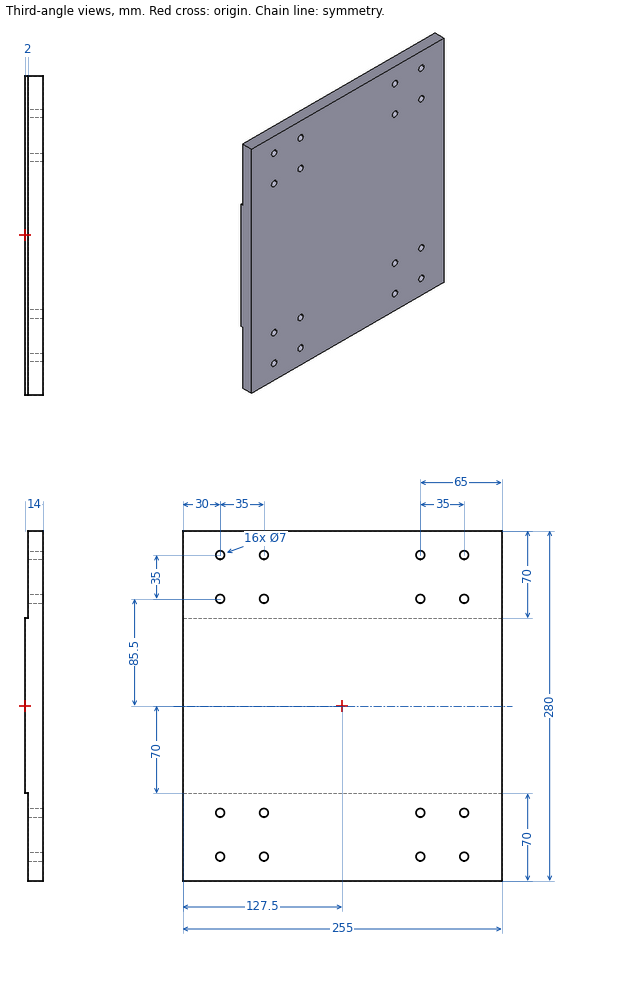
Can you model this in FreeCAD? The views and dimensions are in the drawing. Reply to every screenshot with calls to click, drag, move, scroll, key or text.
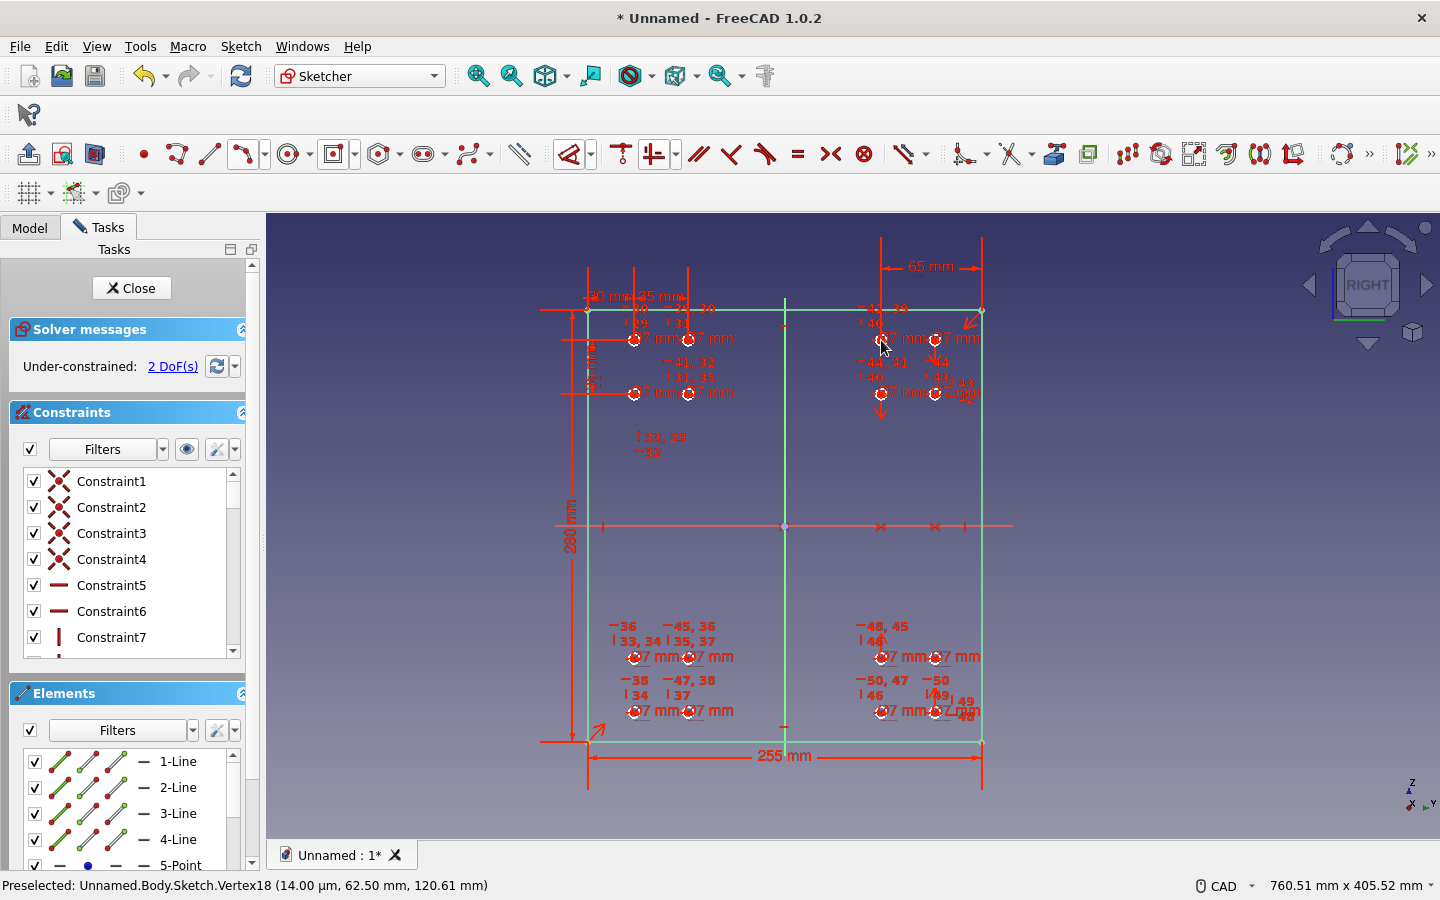
click(935, 340)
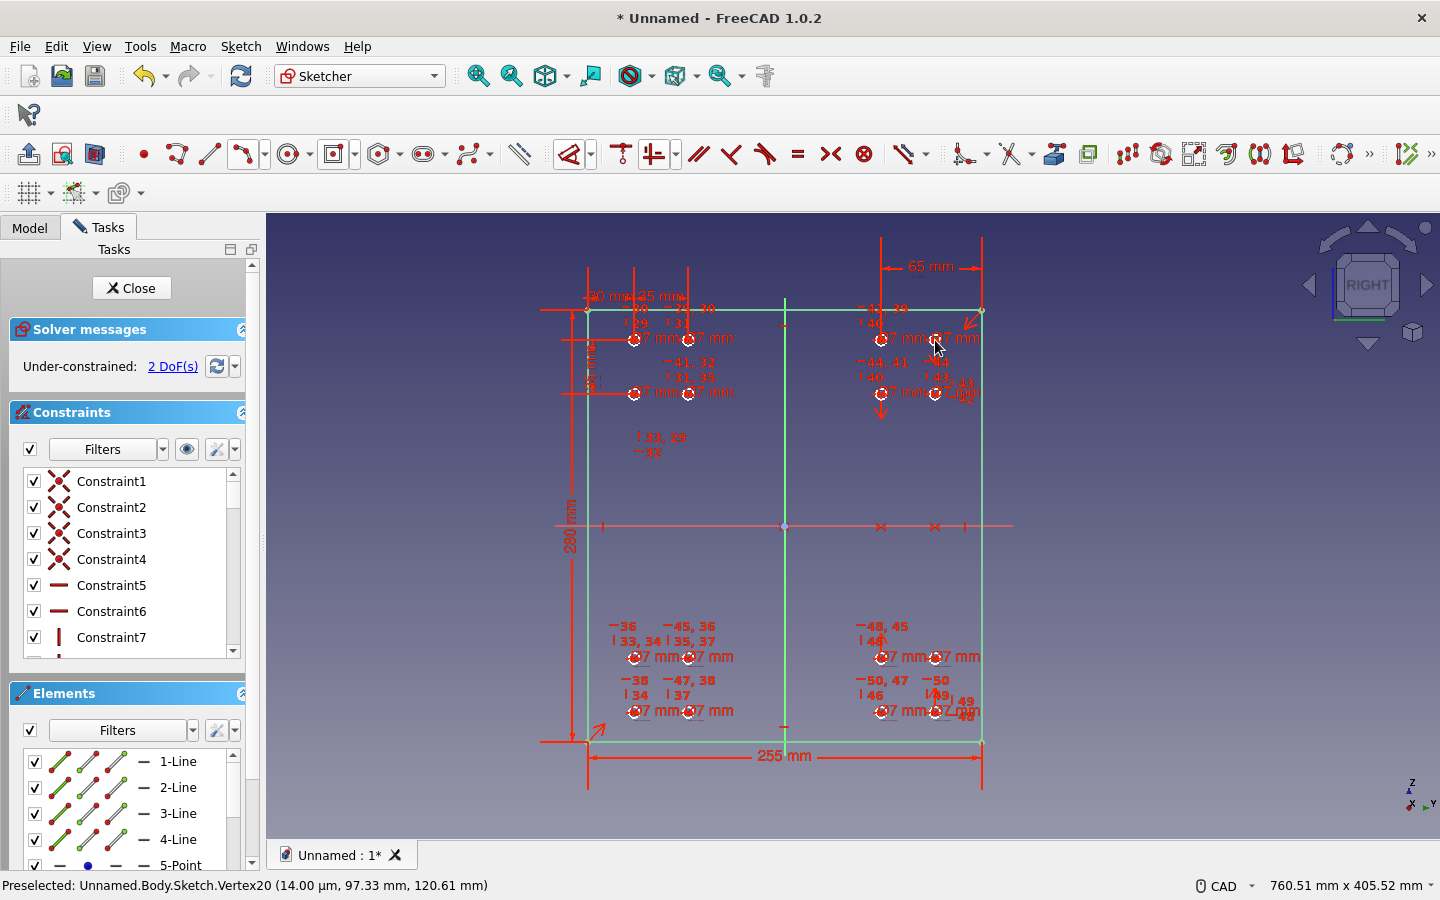
click(590, 154)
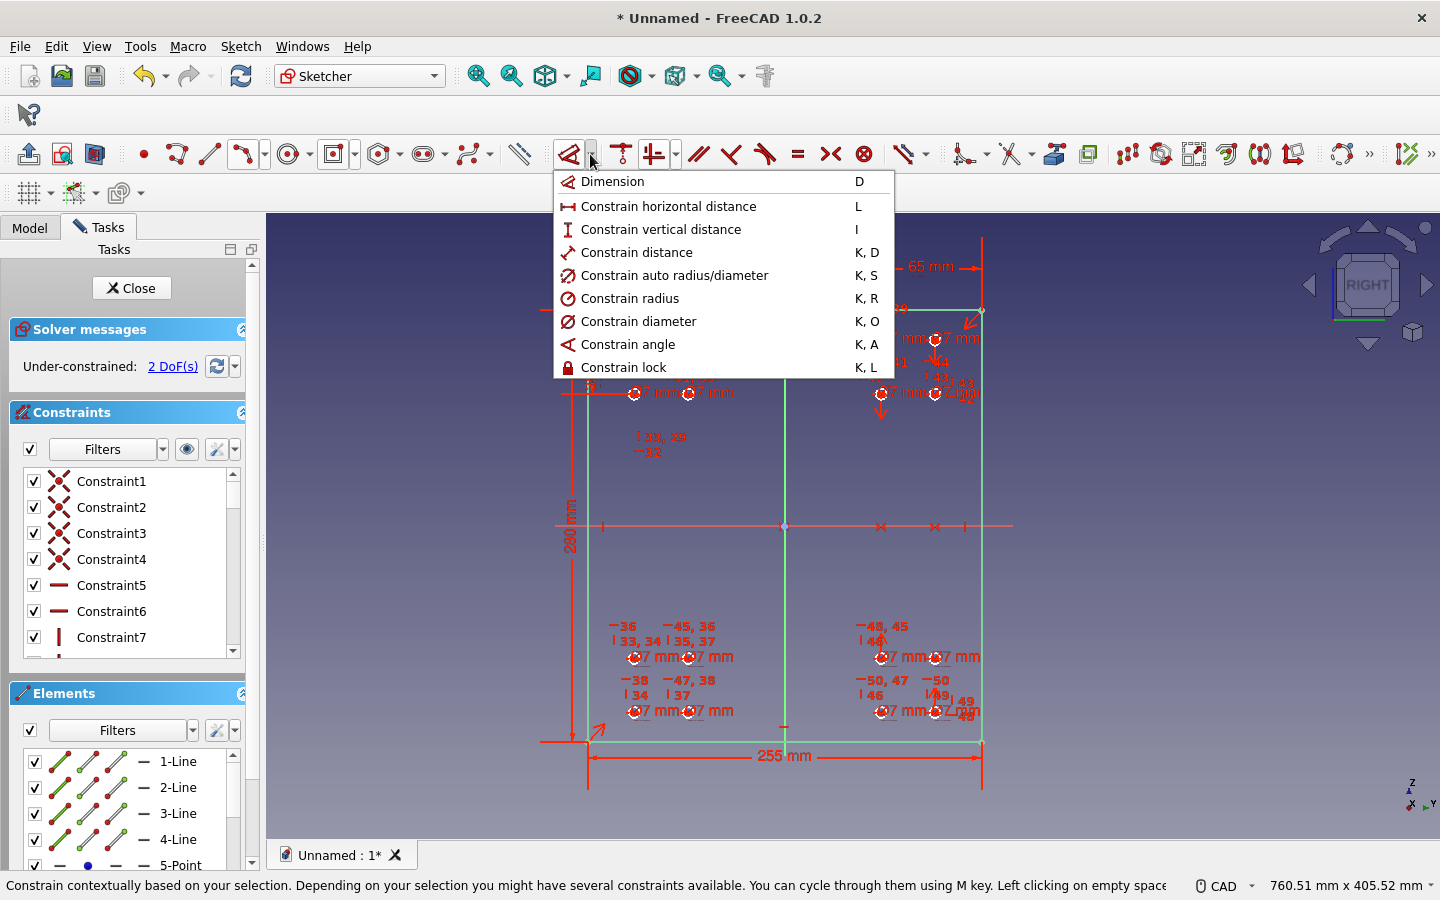
click(724, 206)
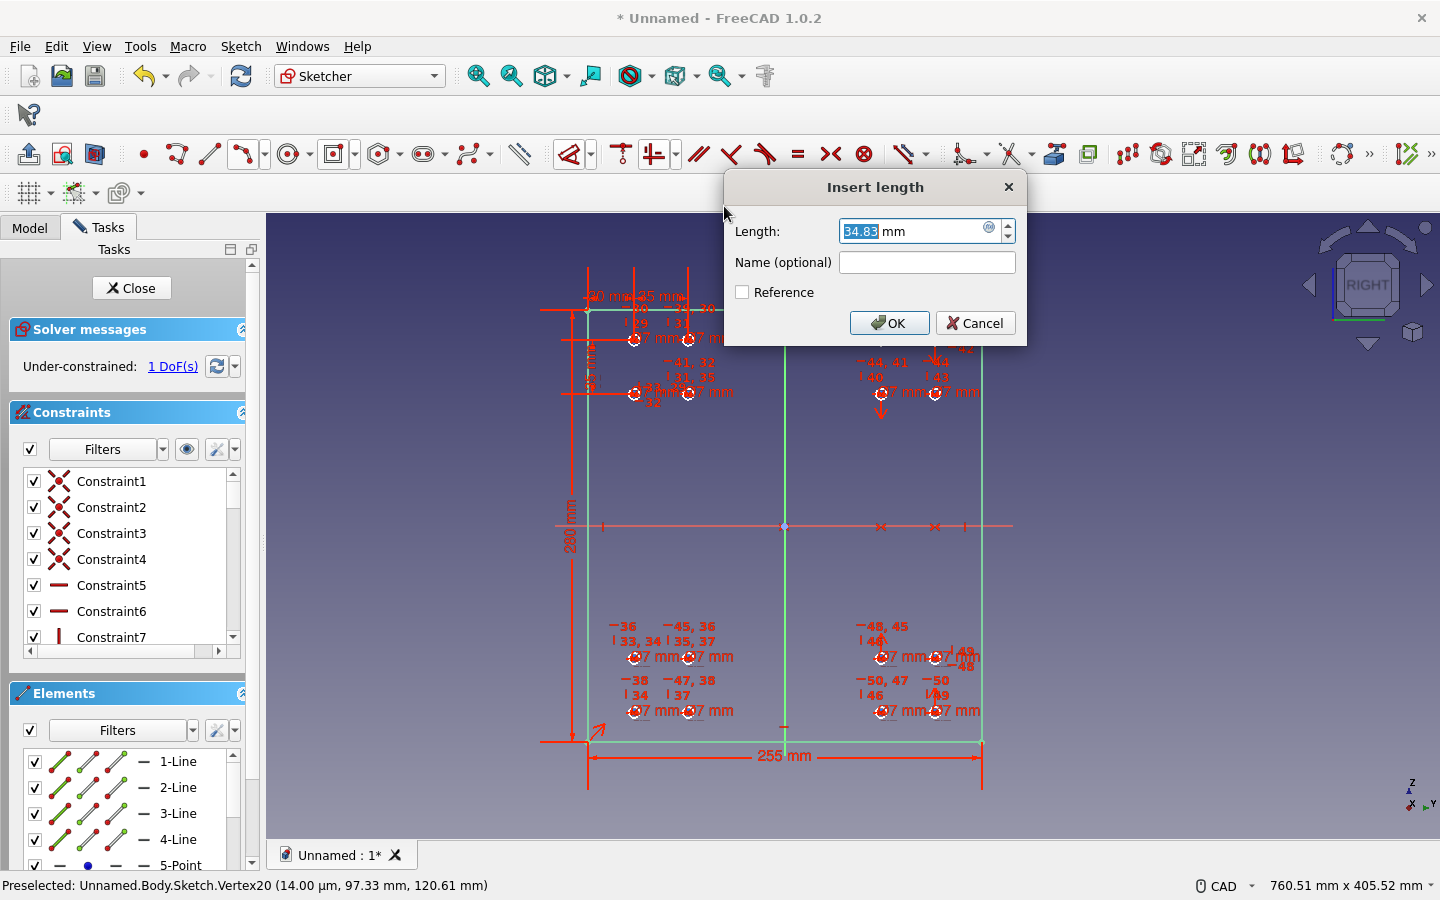
text(35)
key(Return)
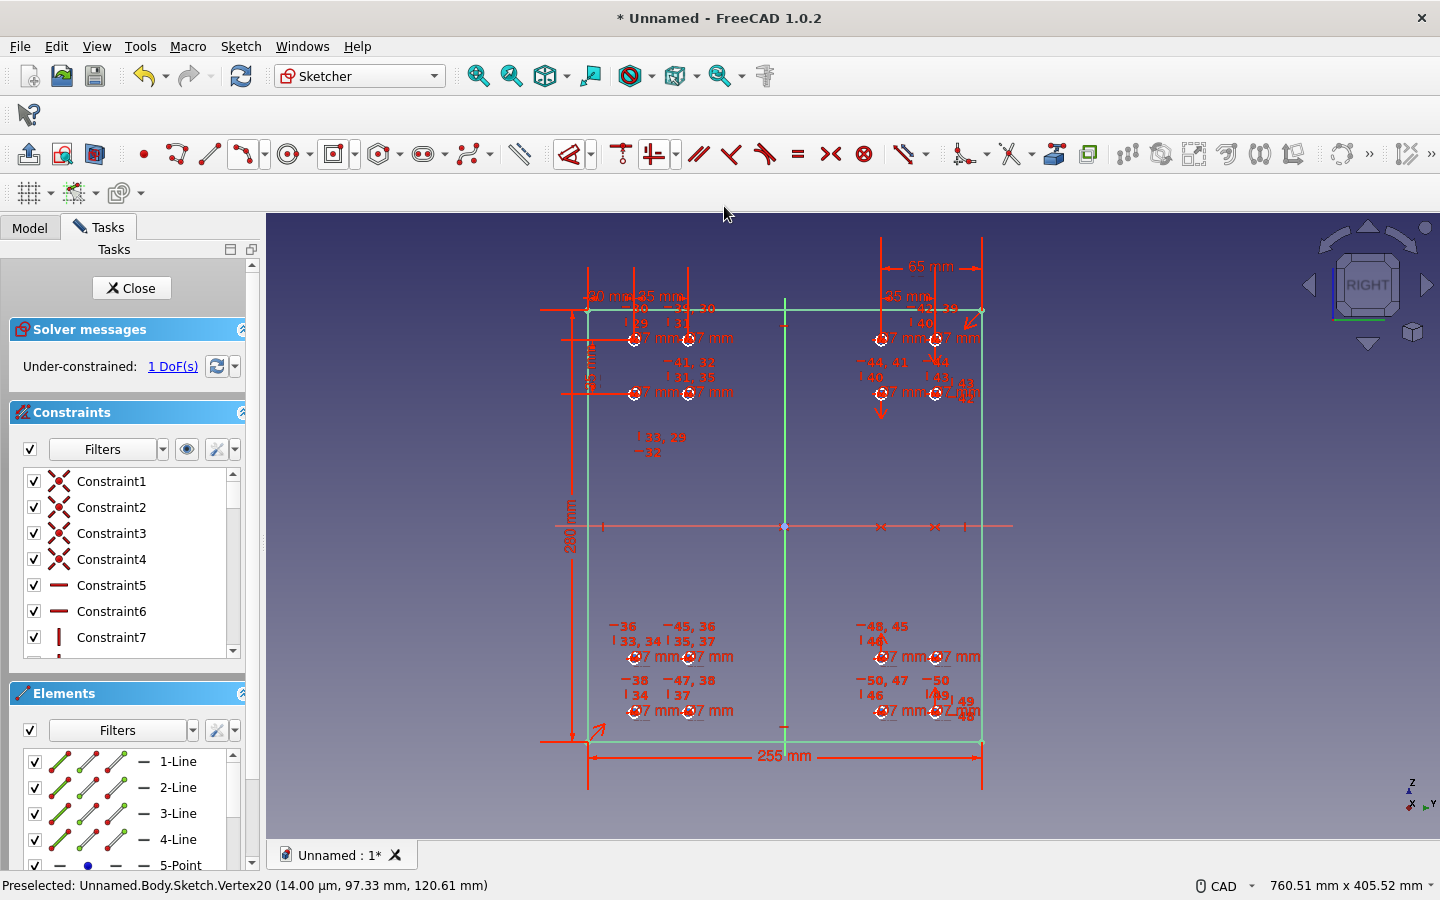
click(634, 394)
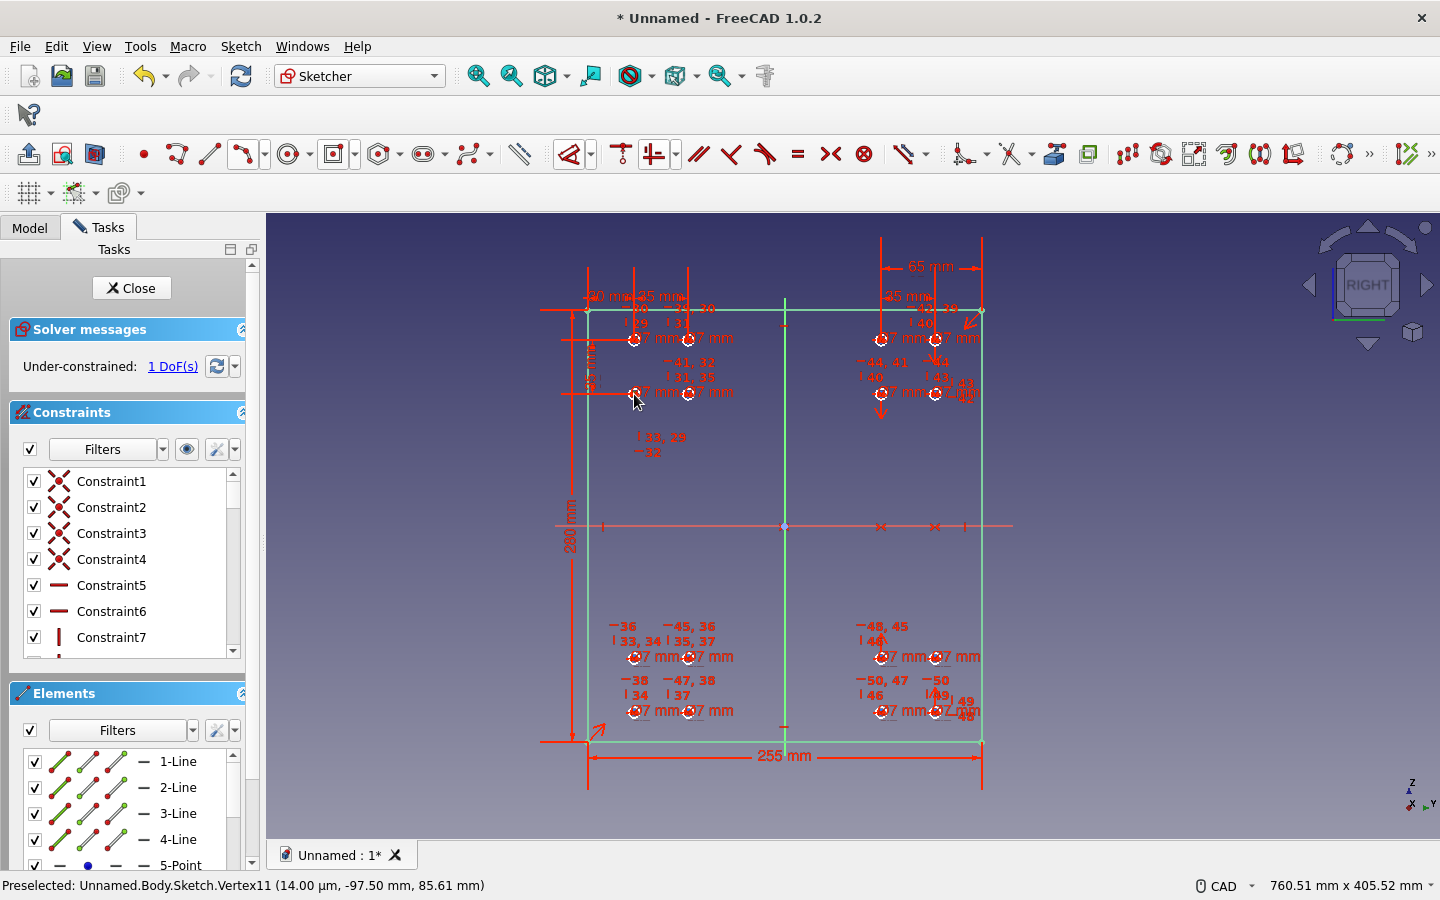
click(590, 154)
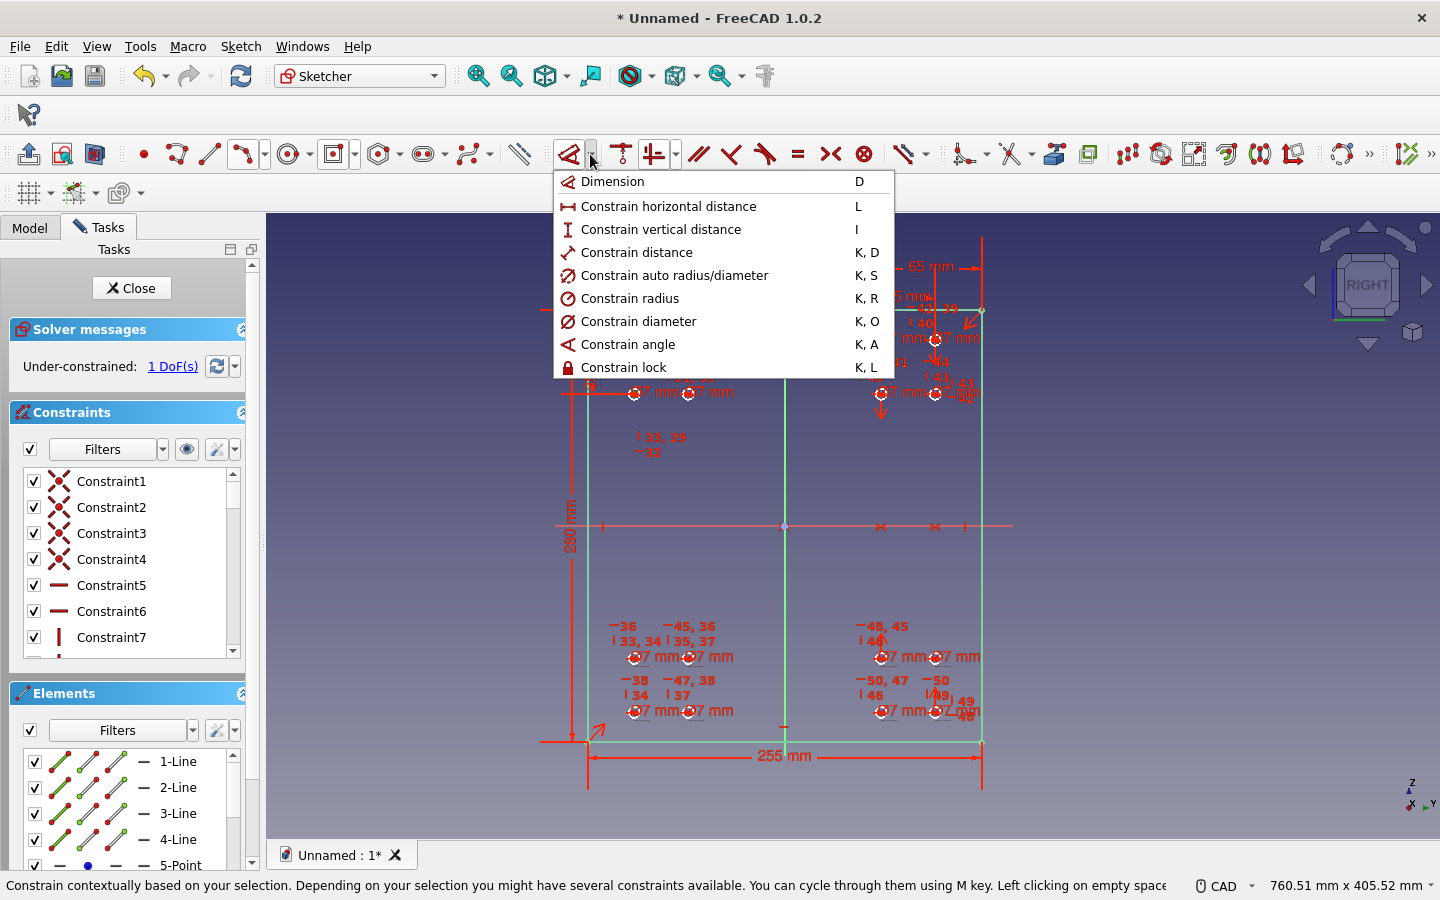
click(724, 230)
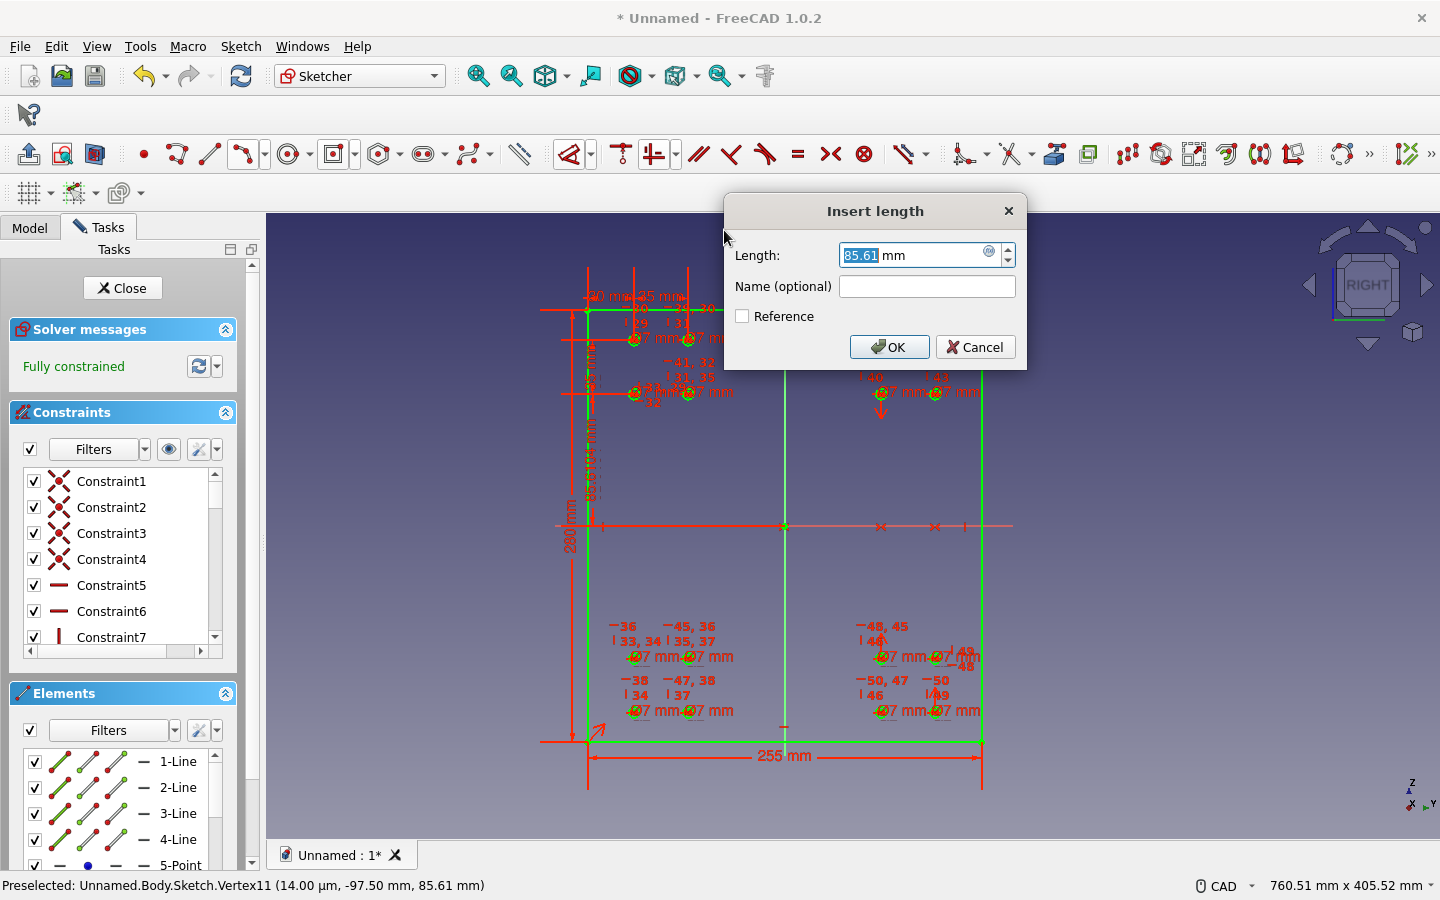
text(85.5)
key(Return)